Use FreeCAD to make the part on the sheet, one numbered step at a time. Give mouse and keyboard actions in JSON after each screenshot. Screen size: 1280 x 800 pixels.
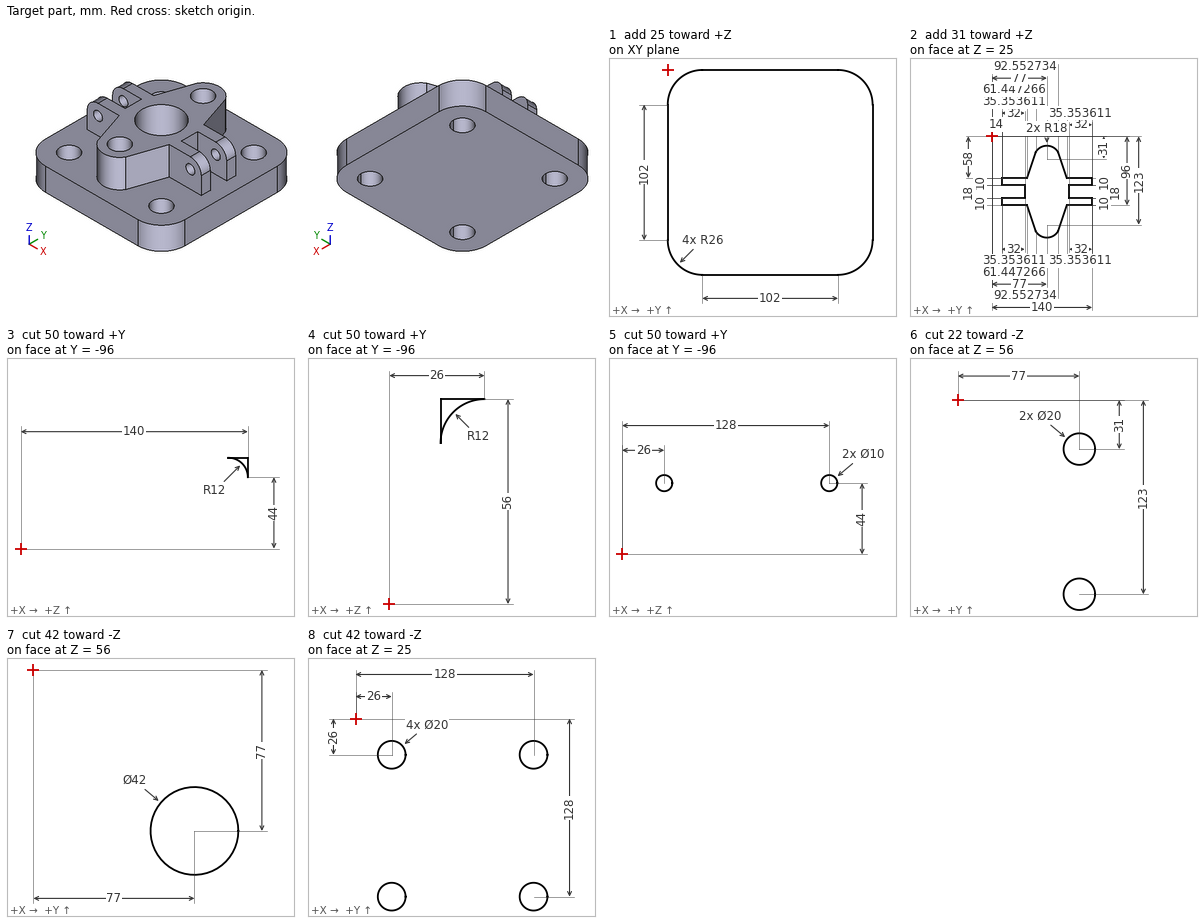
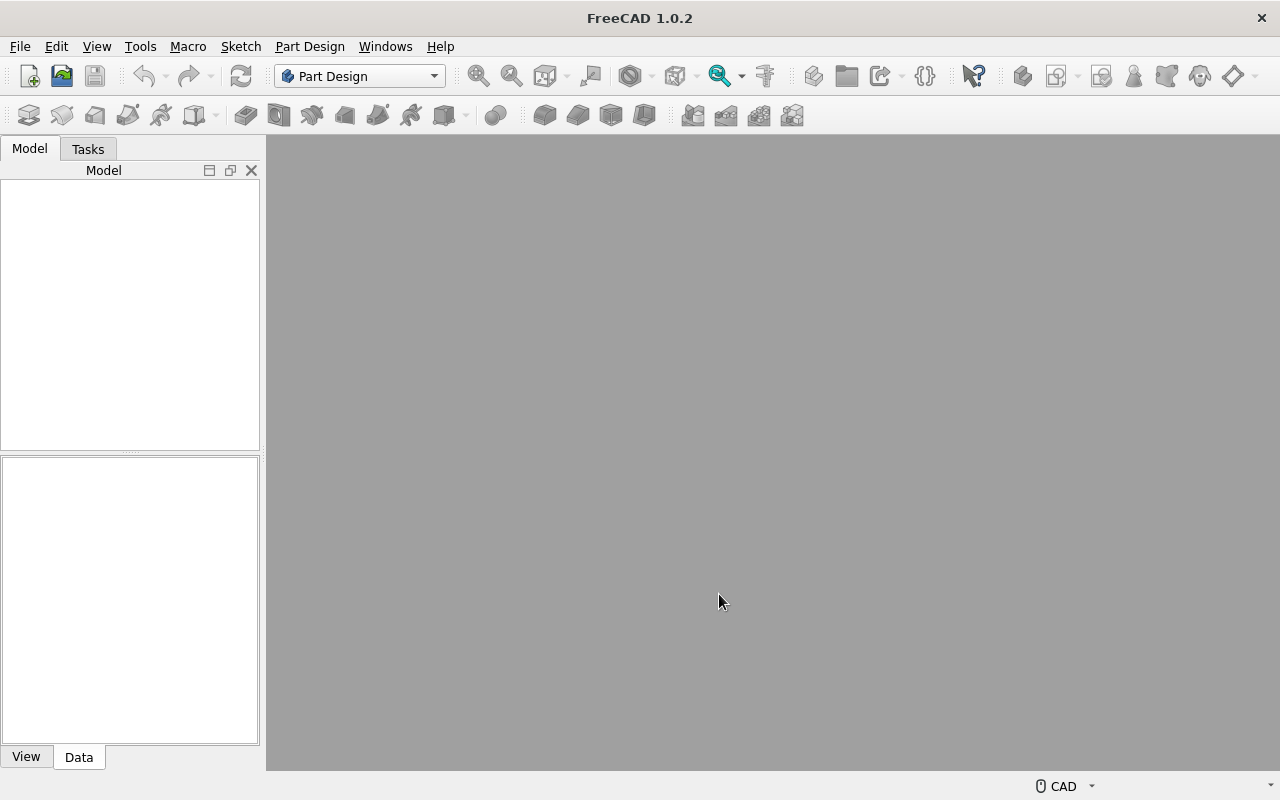
{"action": "left_click", "coordinate": [29, 76]}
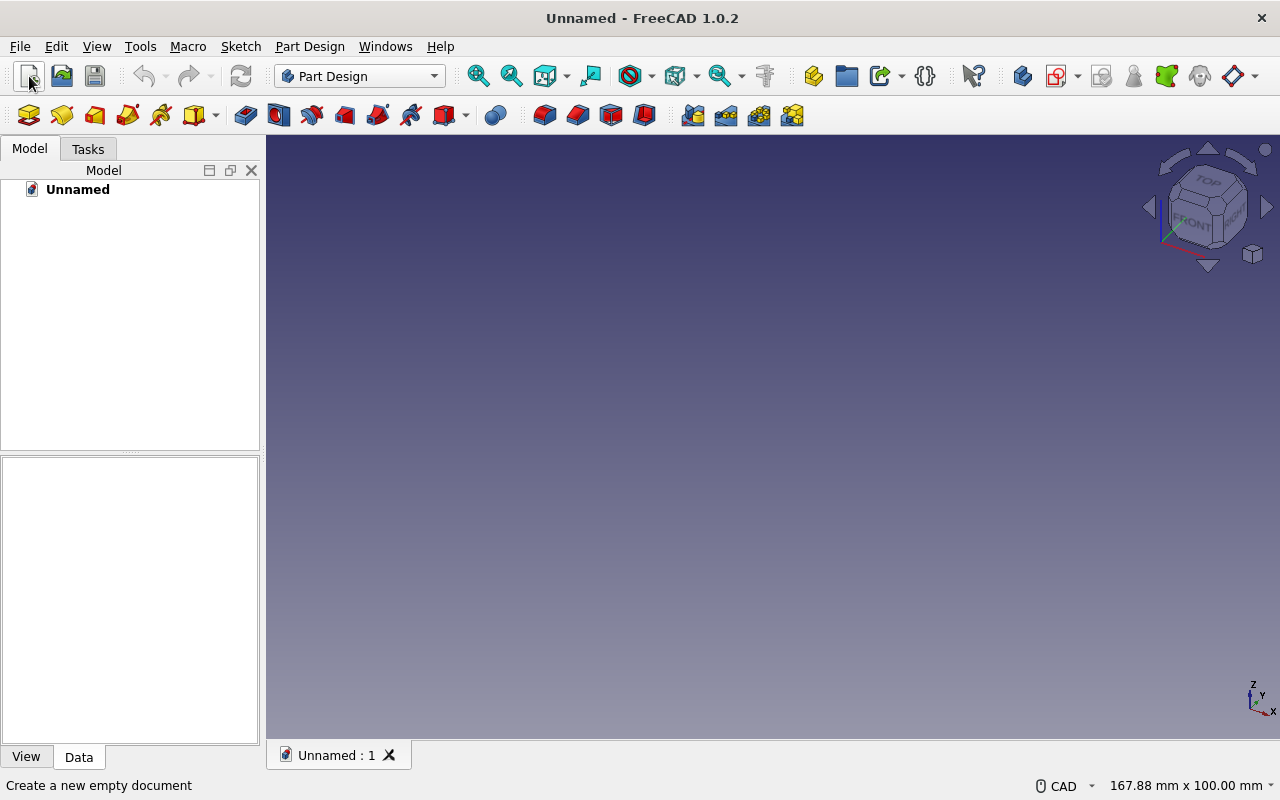
{"action": "left_click", "coordinate": [1056, 76]}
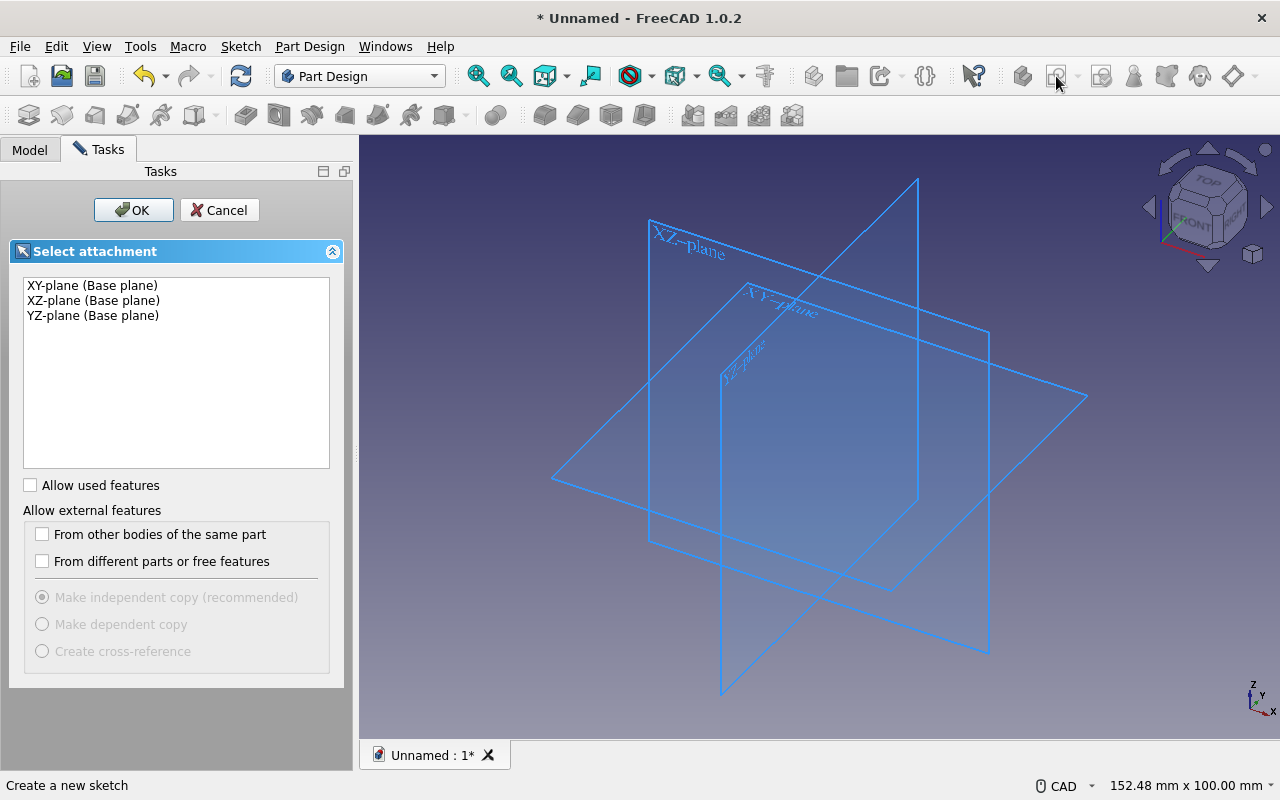
{"action": "left_click", "coordinate": [84, 286]}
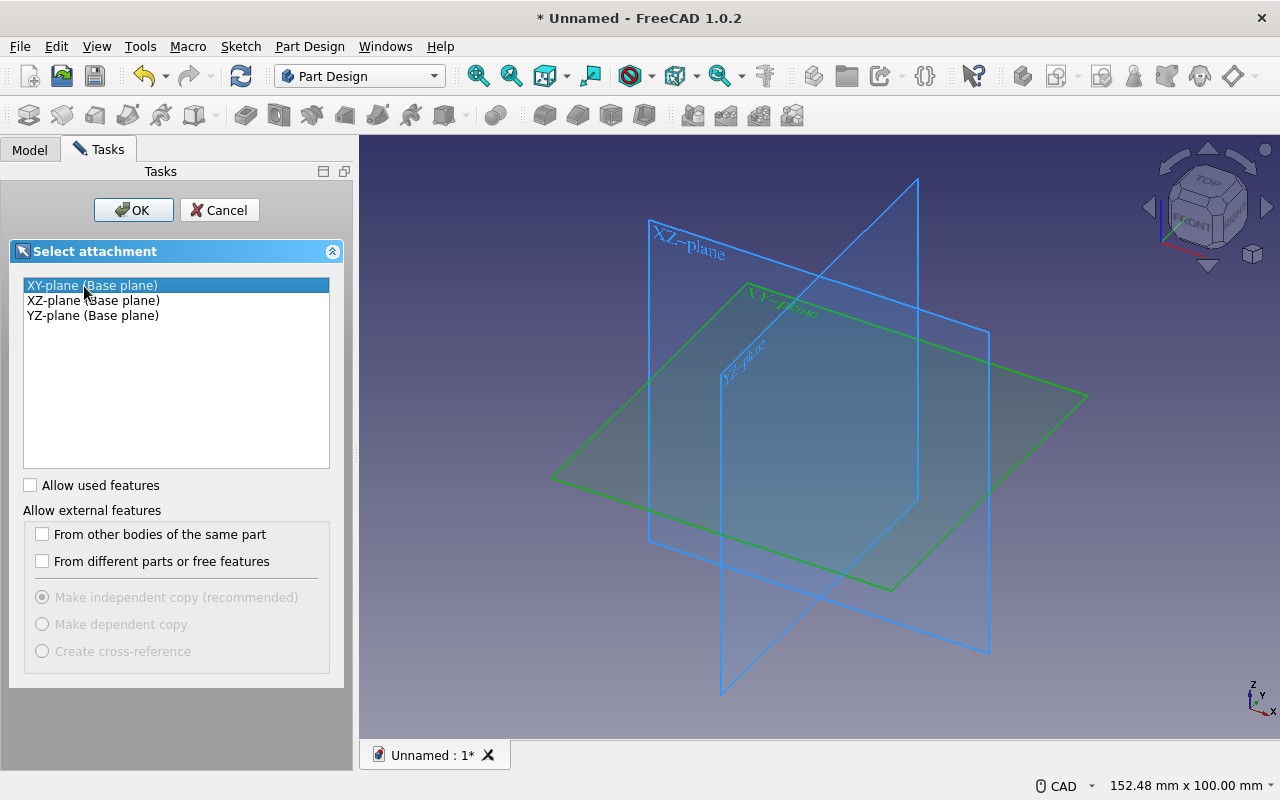
{"action": "left_click", "coordinate": [134, 210]}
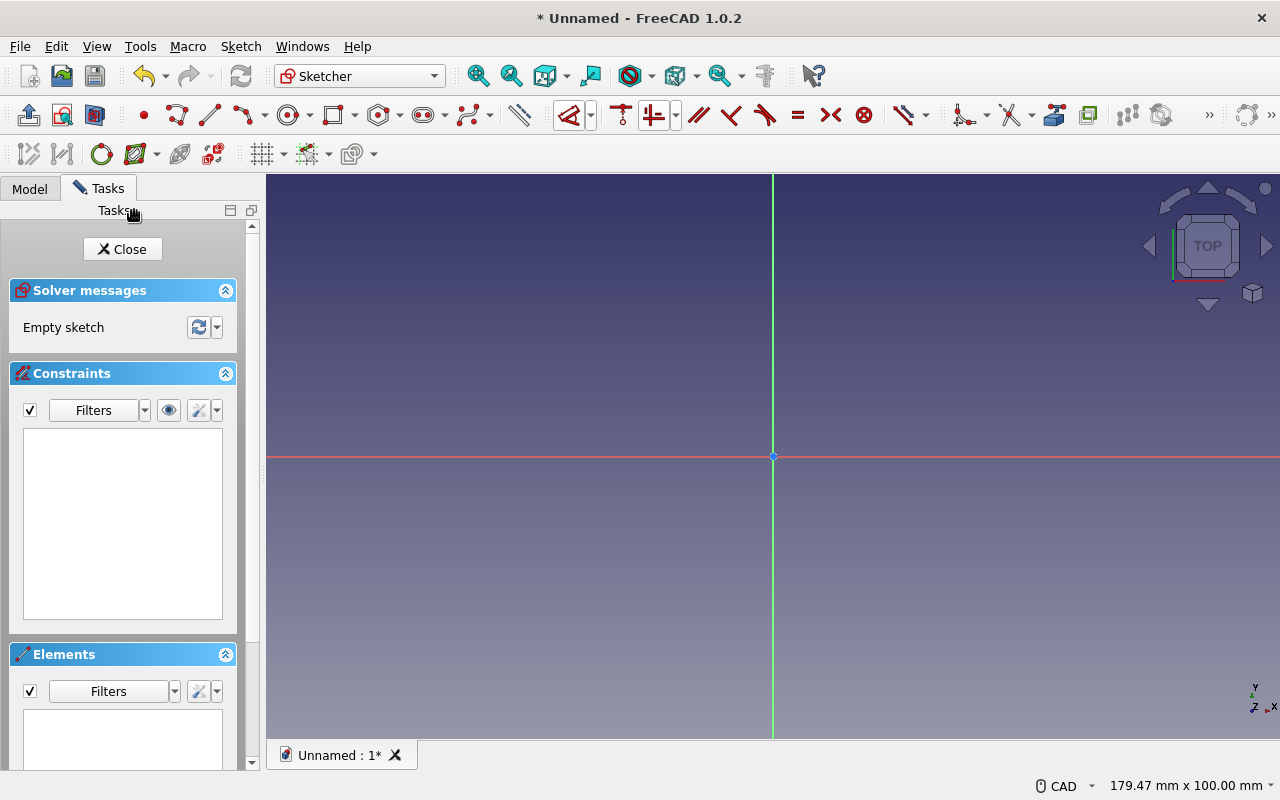
{"action": "scroll", "coordinate": [411, 203], "scroll_direction": "down", "scroll_amount": 5}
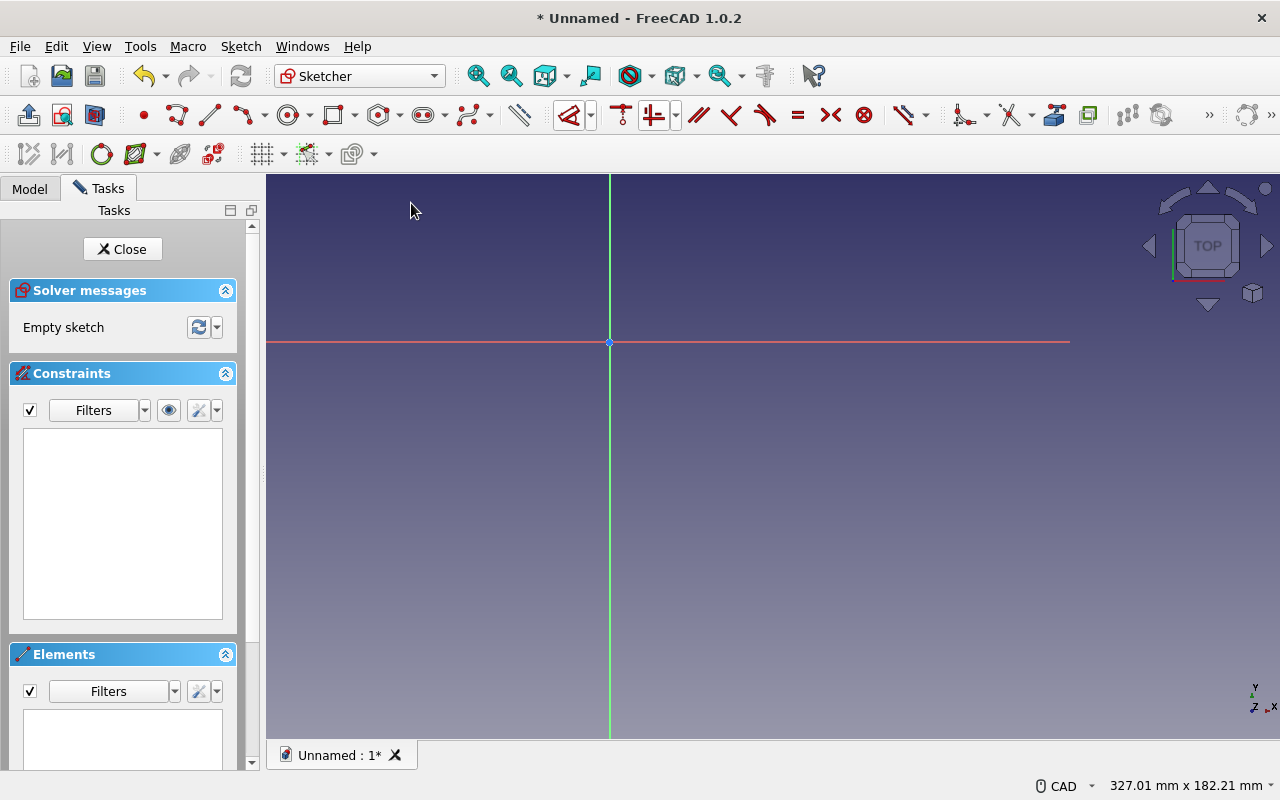
{"action": "left_click", "coordinate": [210, 116]}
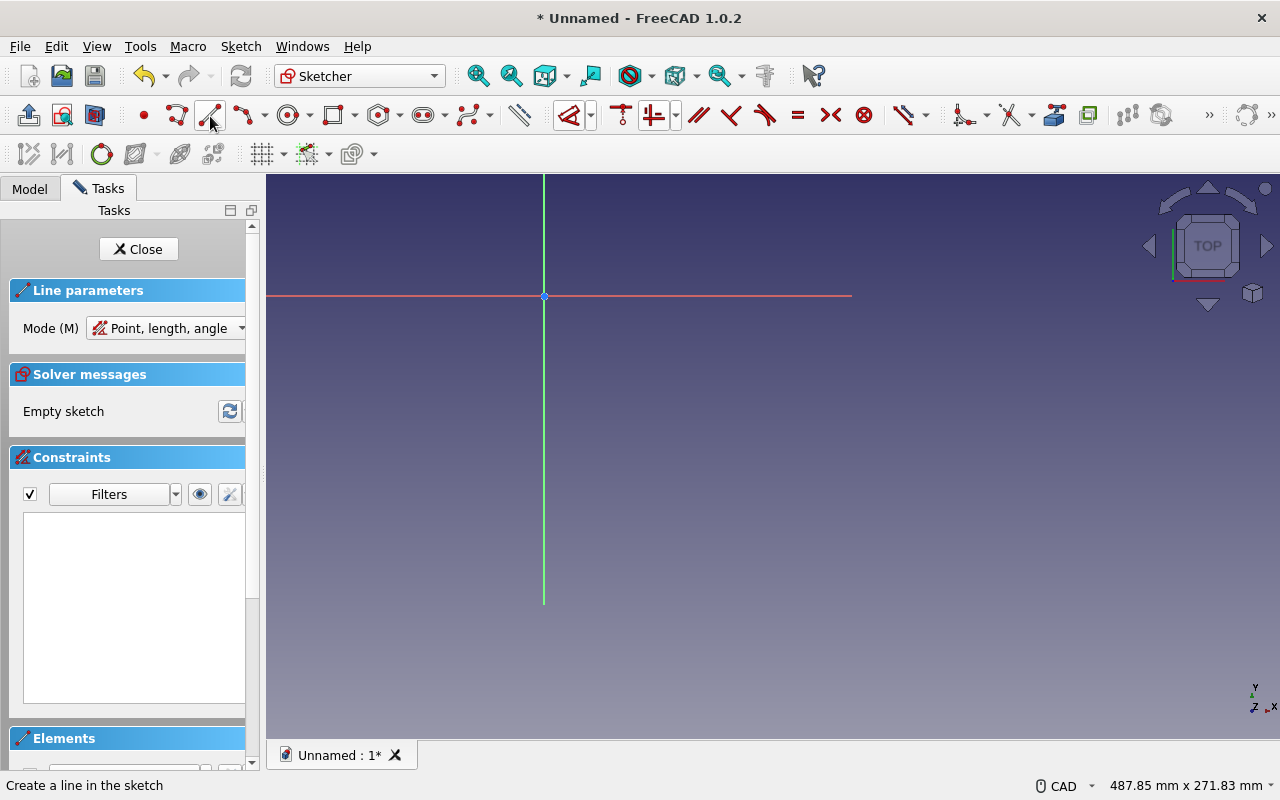
{"action": "left_click", "coordinate": [544, 350]}
{"action": "left_click", "coordinate": [553, 562]}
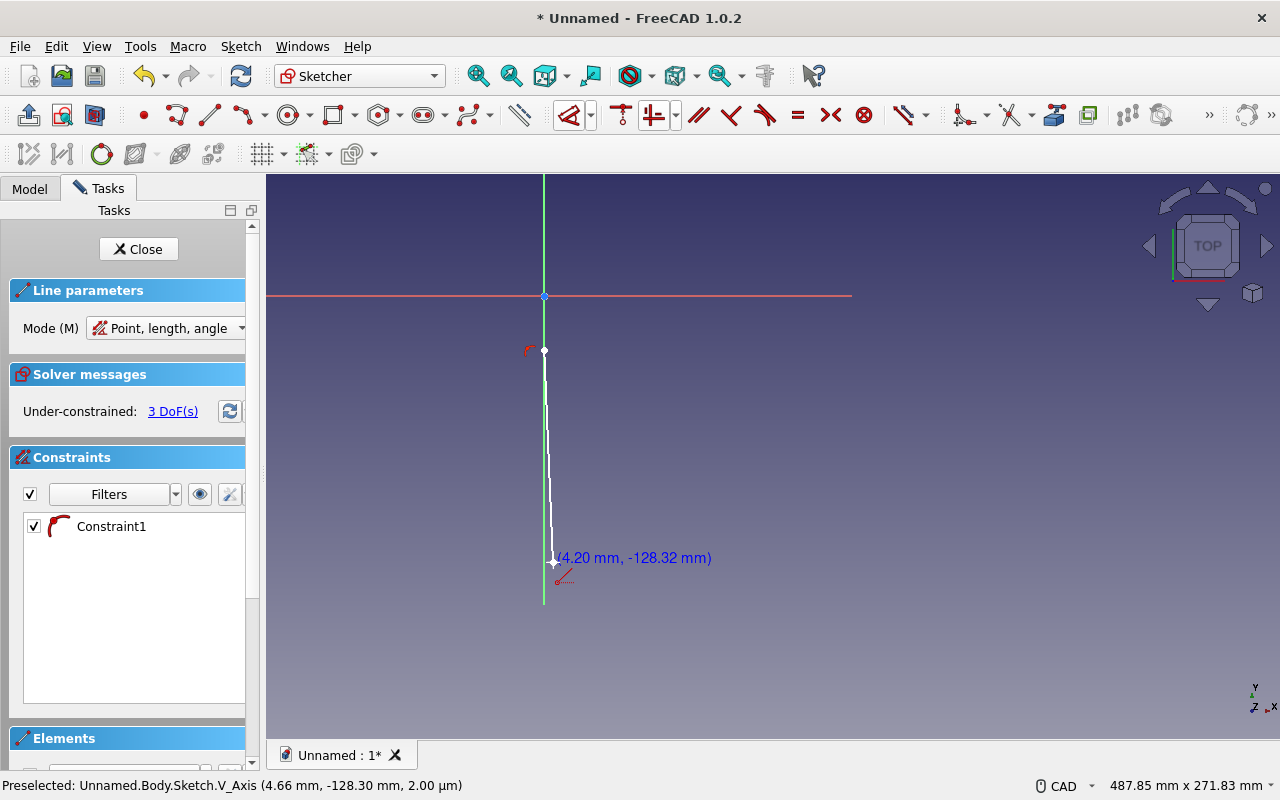
{"action": "left_click", "coordinate": [598, 616]}
{"action": "left_click", "coordinate": [810, 616]}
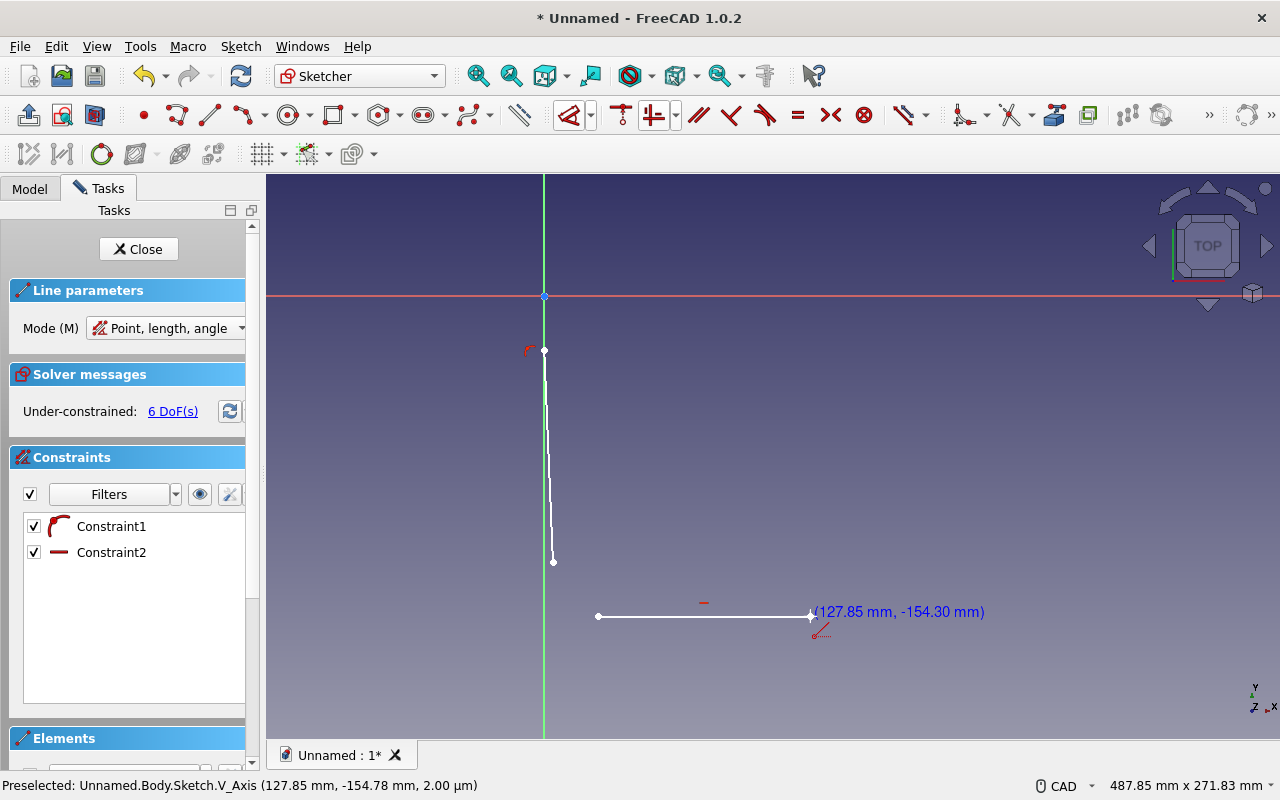
{"action": "left_click", "coordinate": [864, 562]}
{"action": "left_click", "coordinate": [864, 350]}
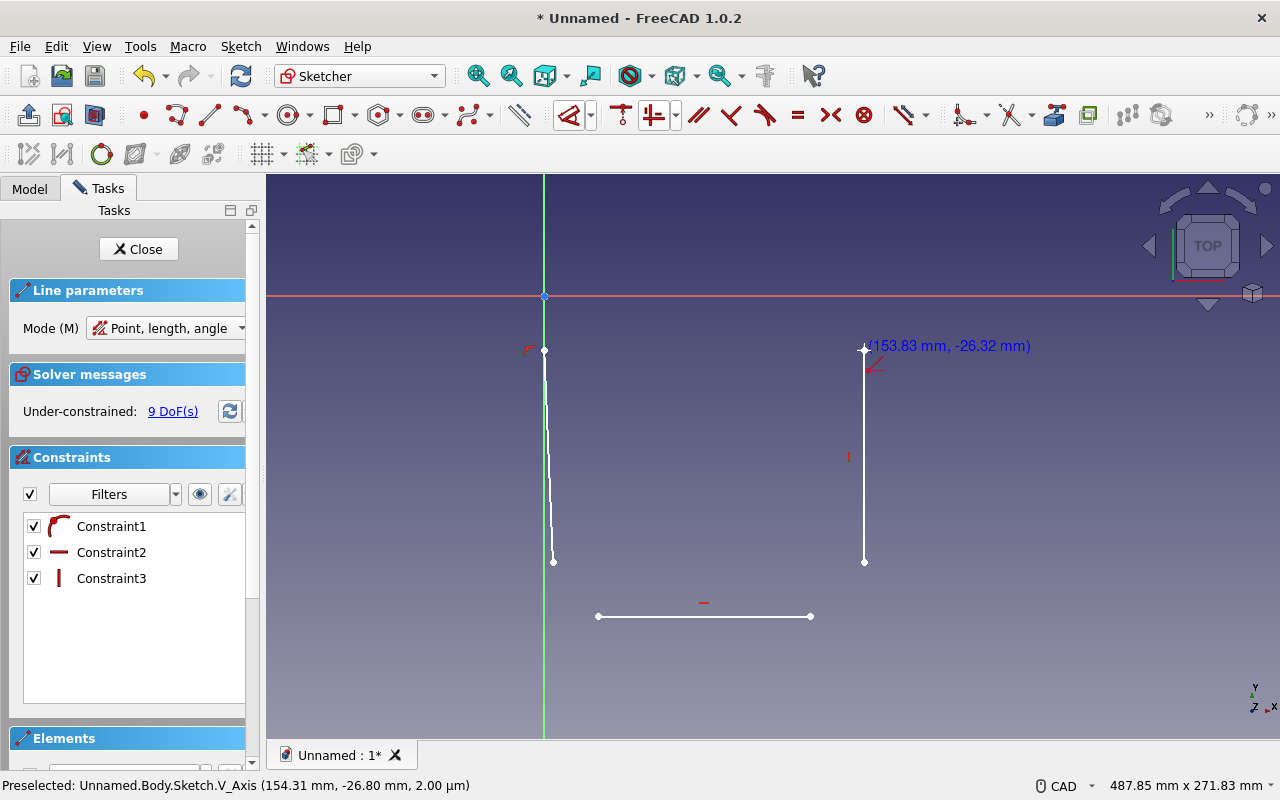
{"action": "left_click", "coordinate": [810, 296]}
{"action": "left_click", "coordinate": [598, 305]}